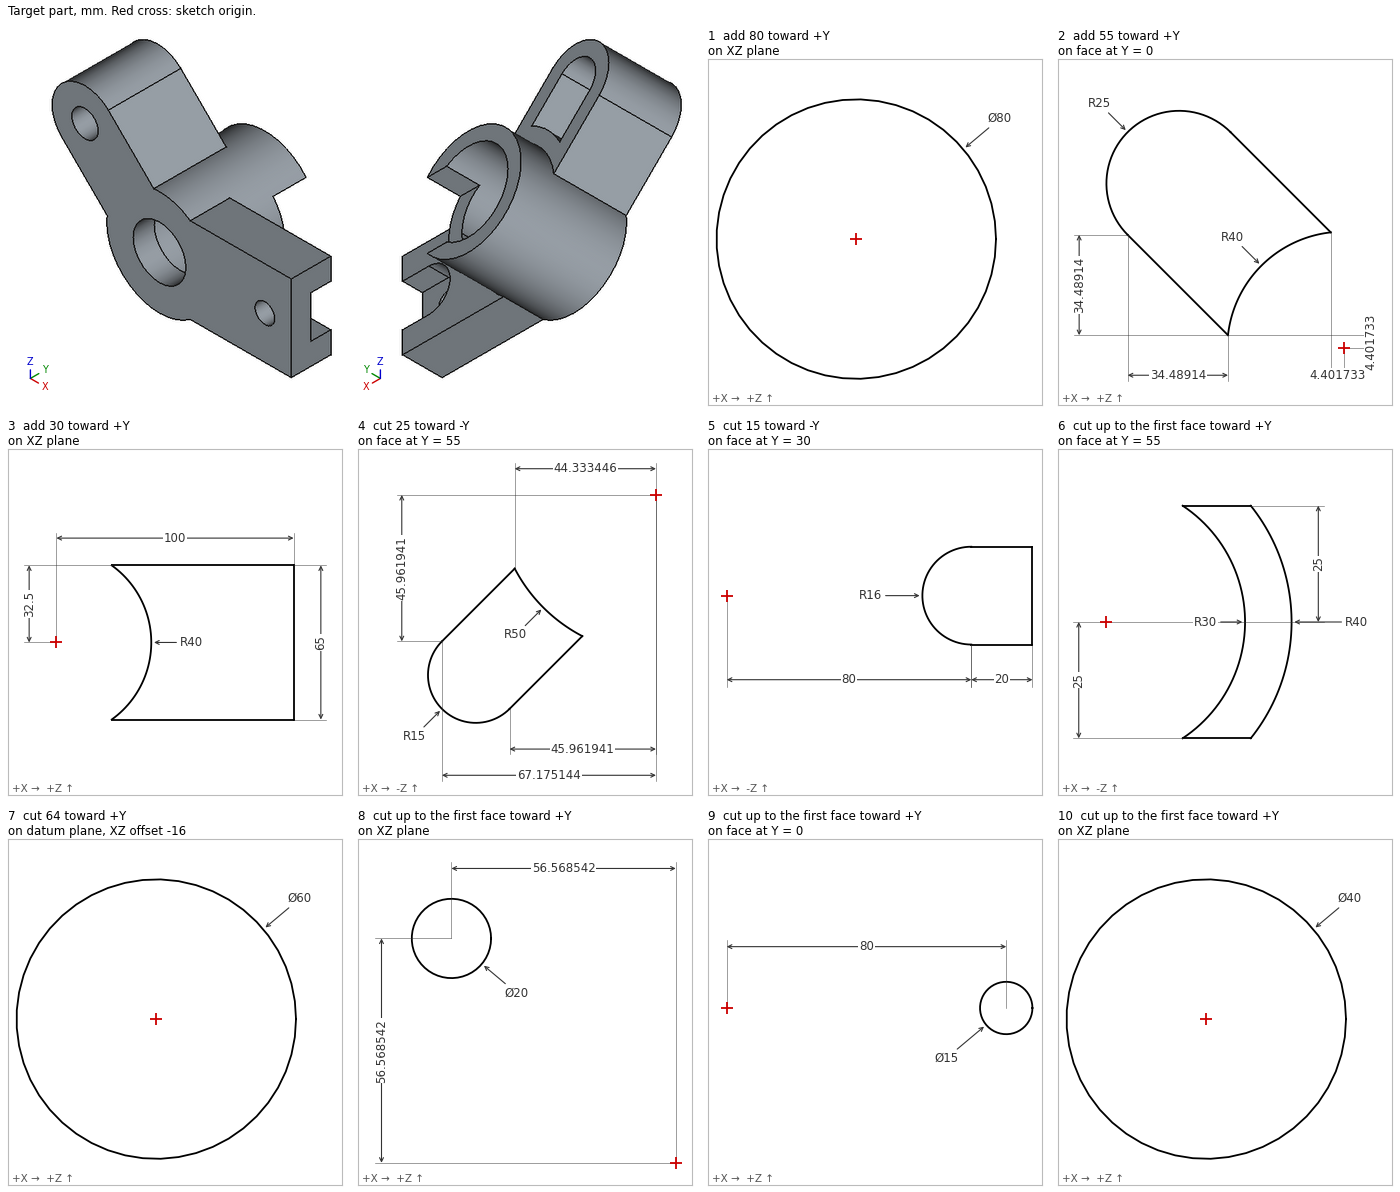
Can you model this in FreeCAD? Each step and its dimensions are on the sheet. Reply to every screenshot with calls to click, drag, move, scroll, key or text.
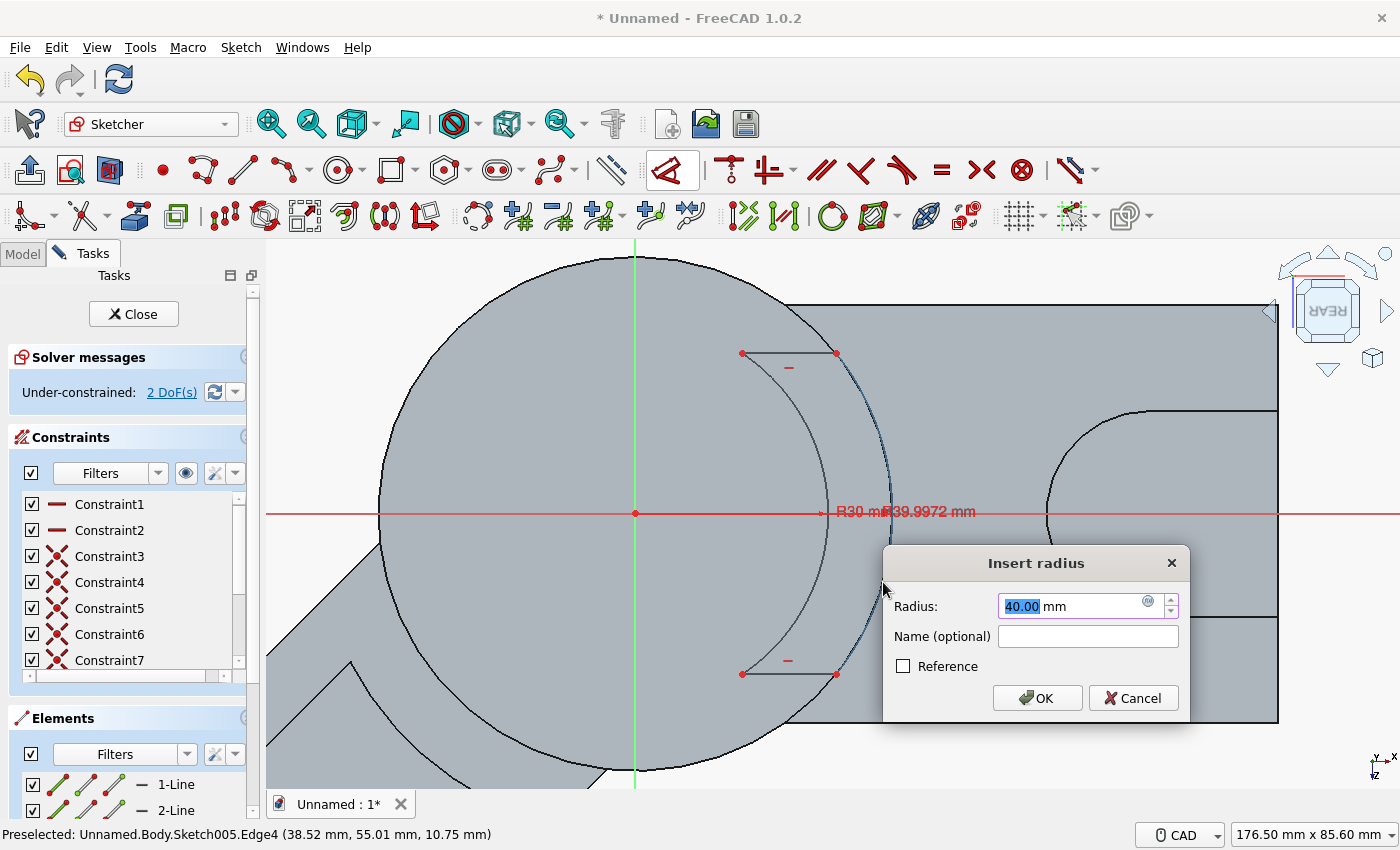
text(40)
key(Return)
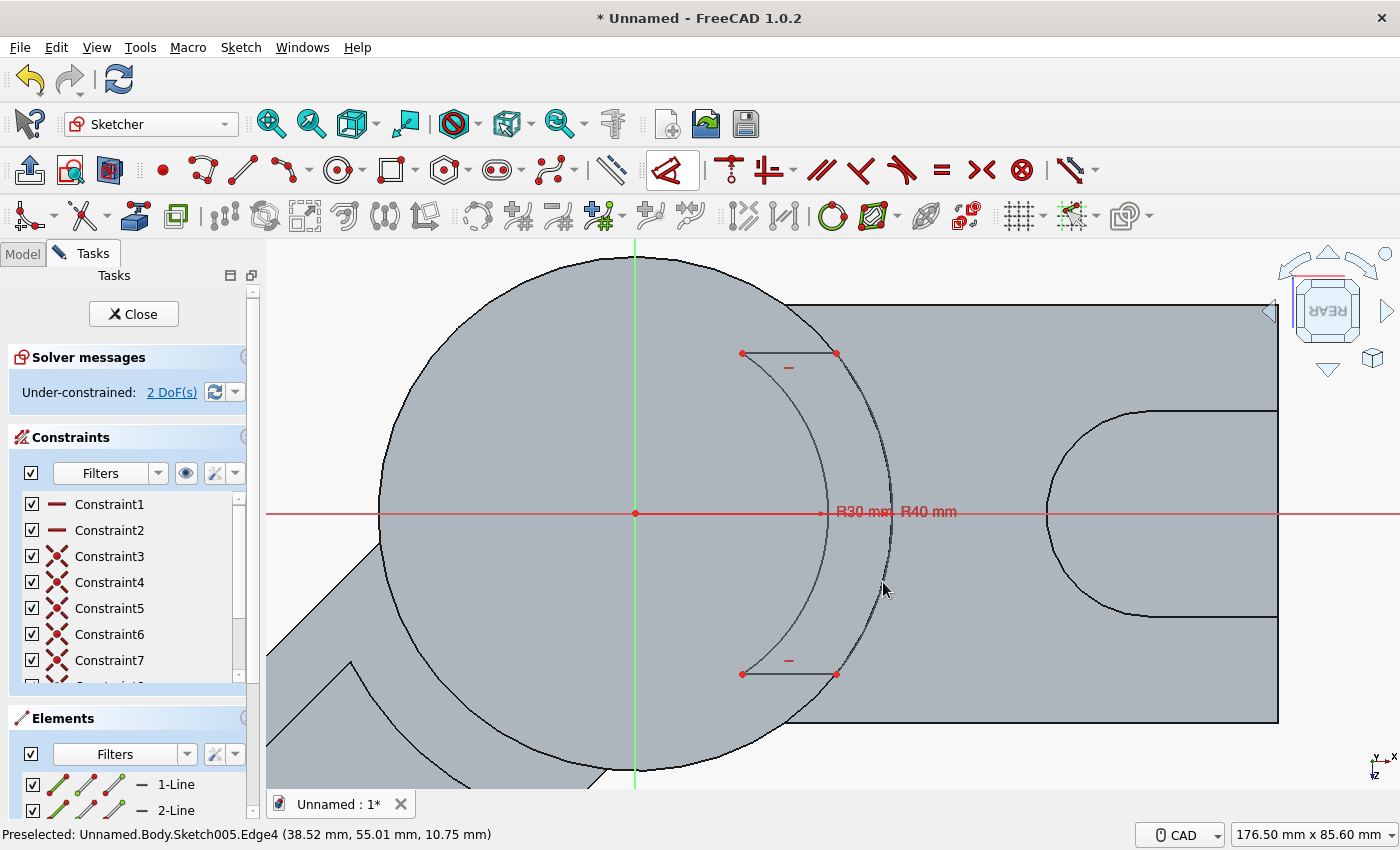
click(836, 353)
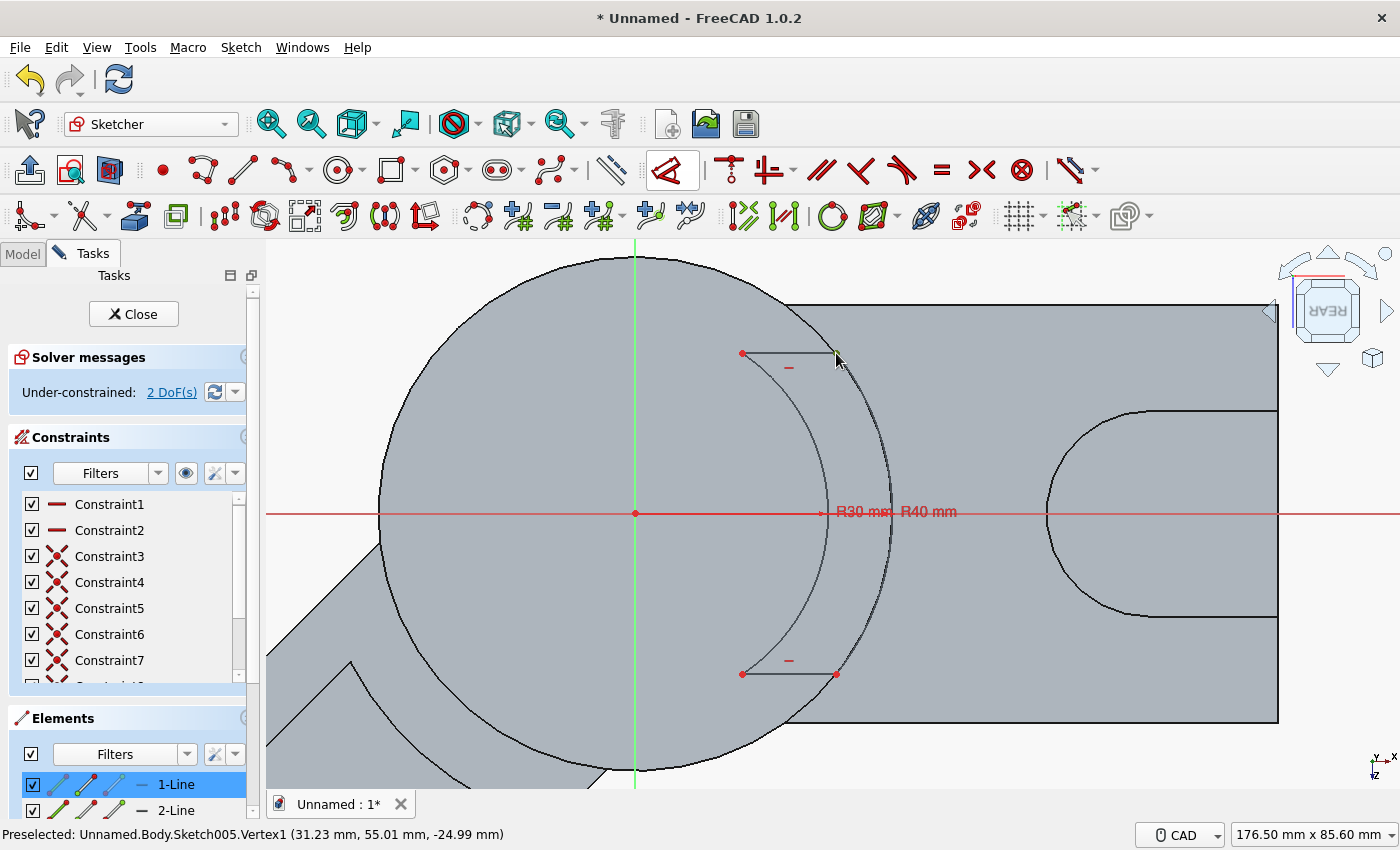
click(694, 170)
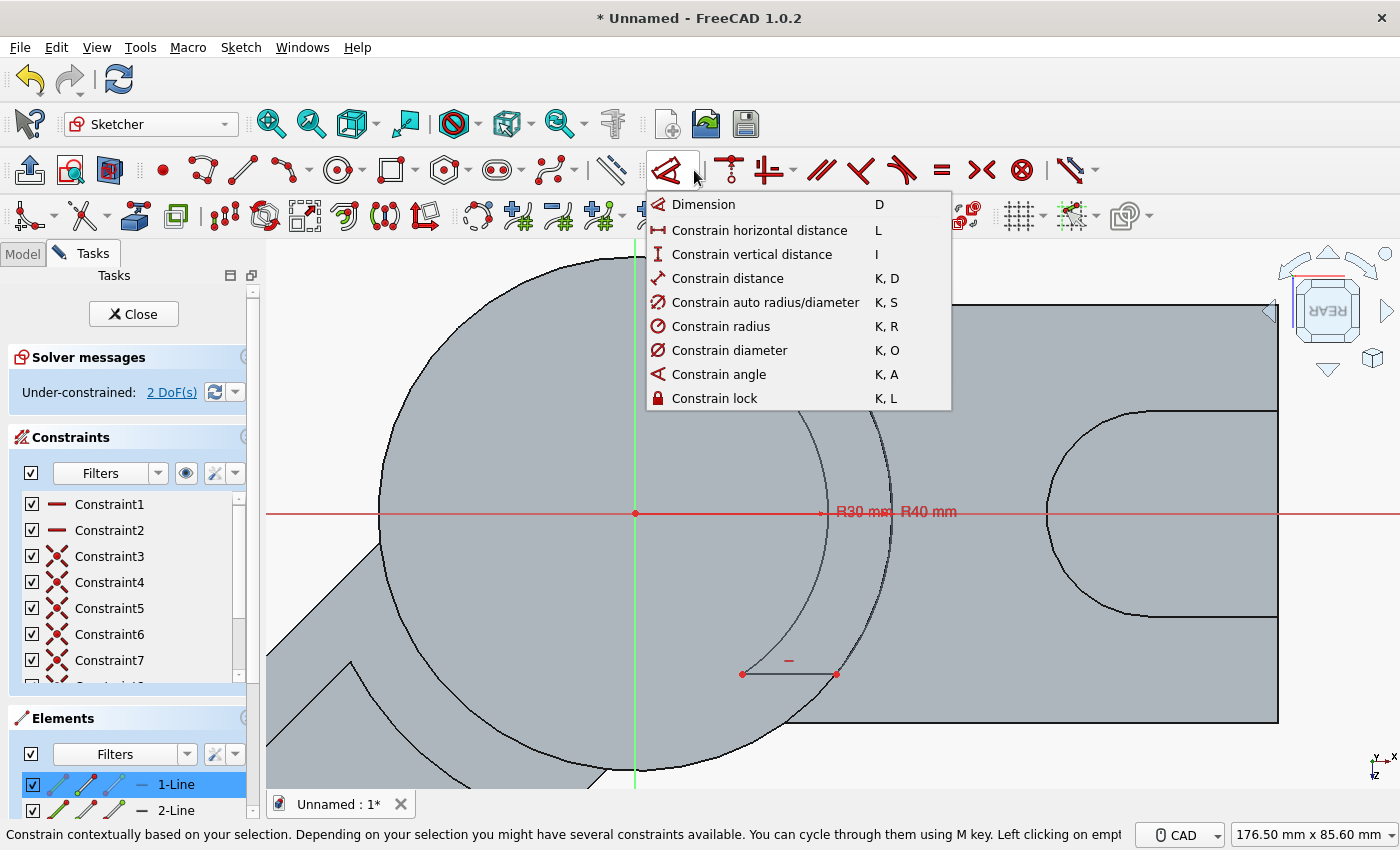
click(799, 254)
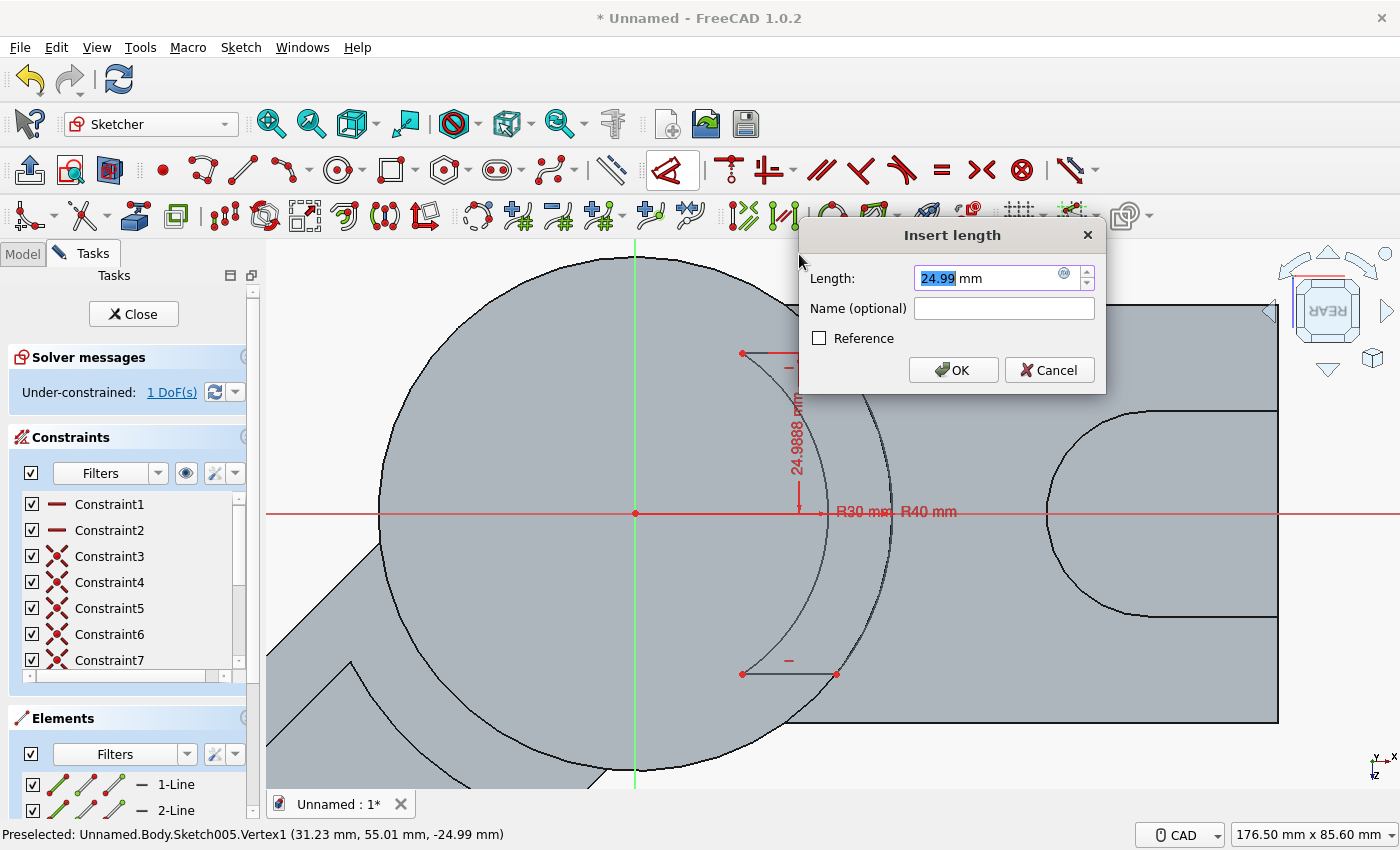
text(25)
key(Return)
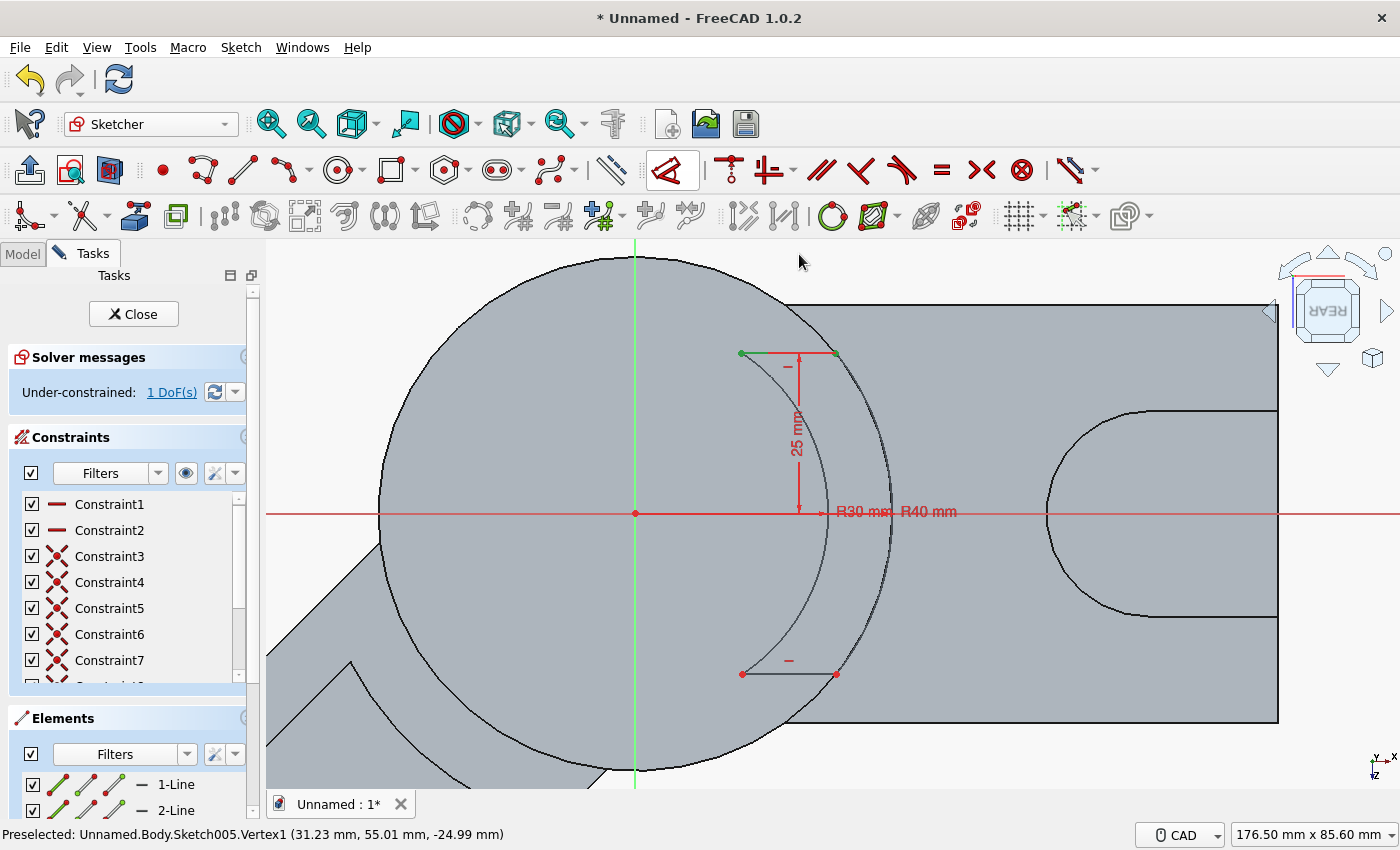
click(742, 674)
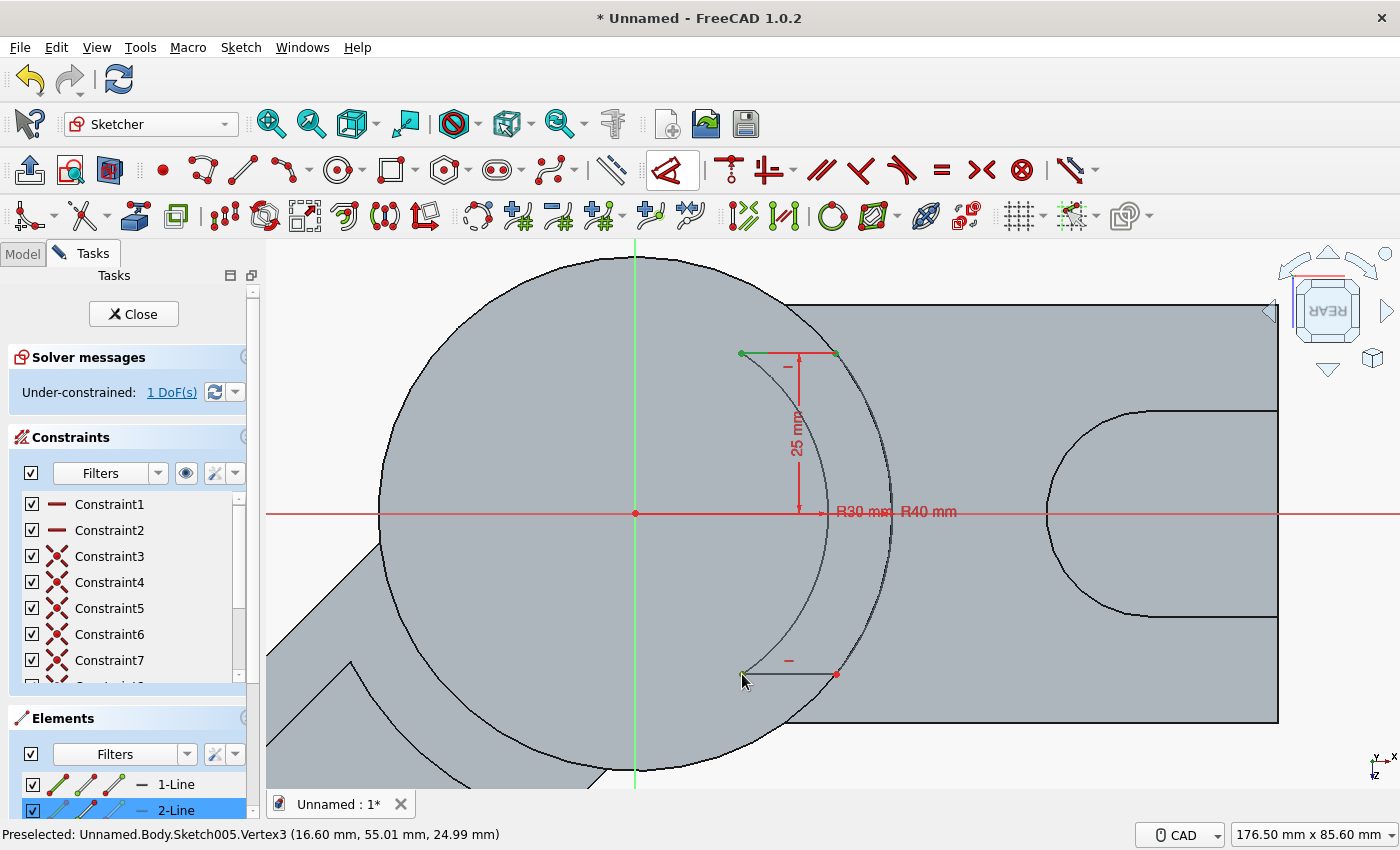
key(i)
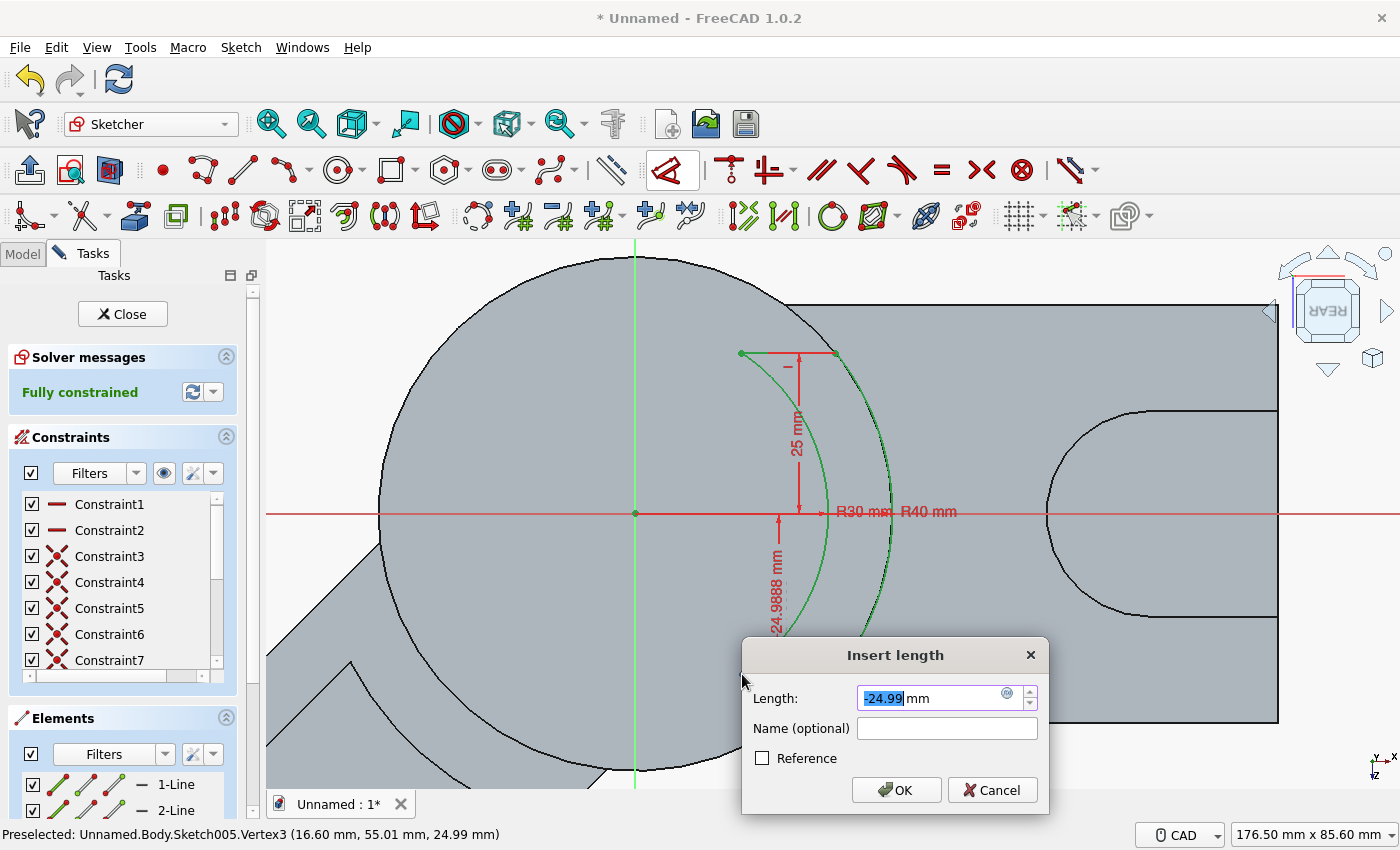
text(-25)
key(Return)